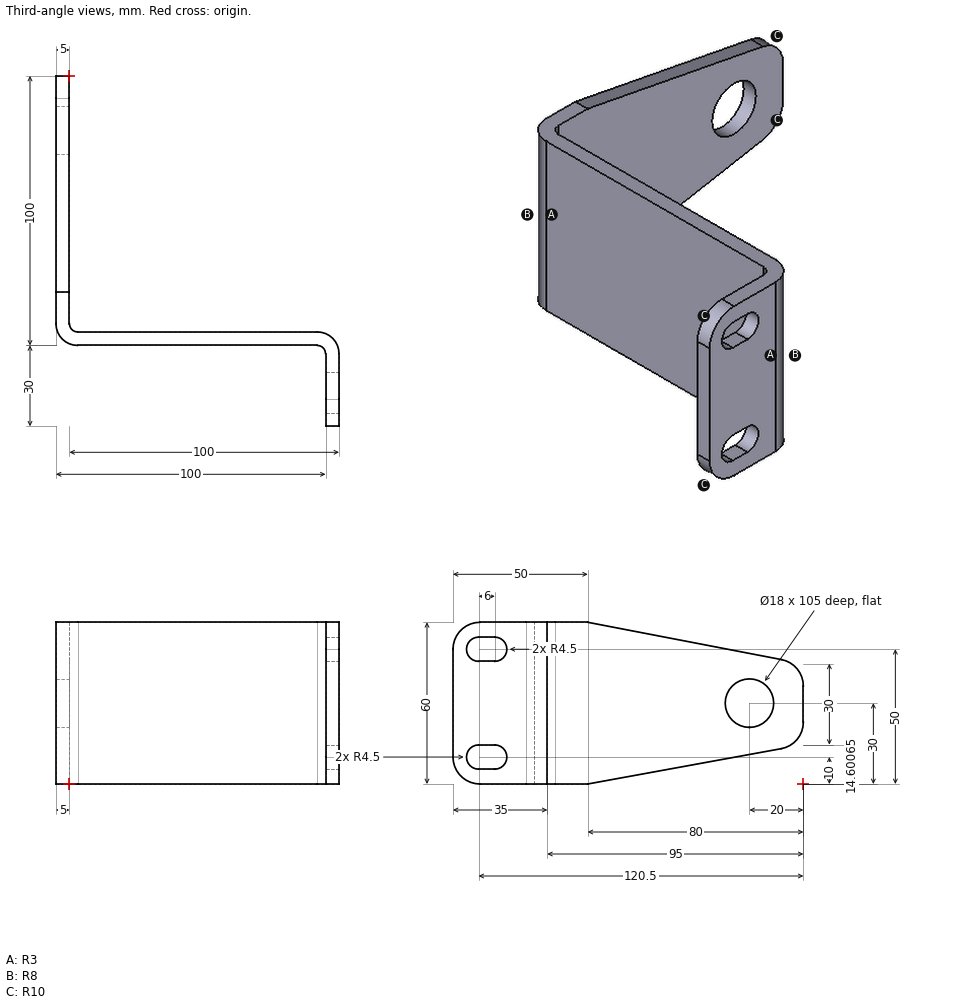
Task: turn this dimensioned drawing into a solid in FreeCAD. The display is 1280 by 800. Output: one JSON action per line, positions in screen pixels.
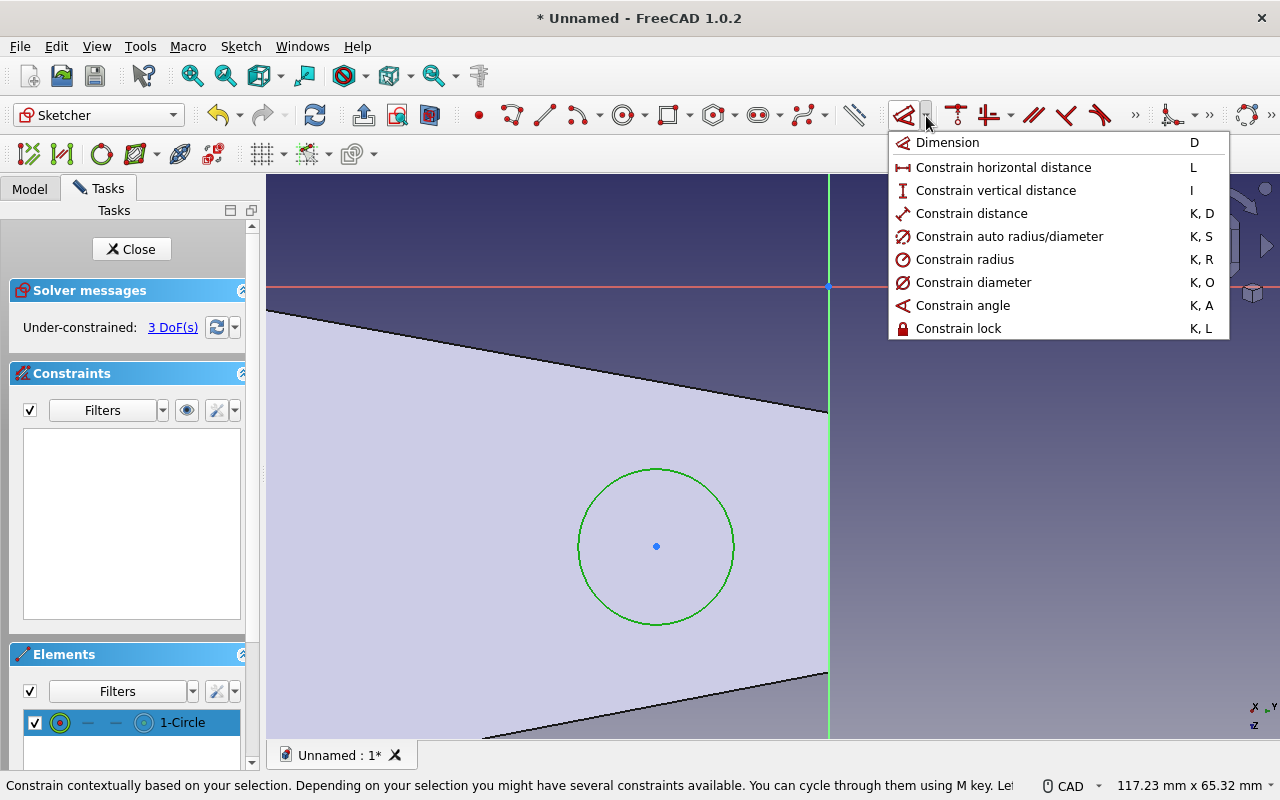
{"action": "left_click", "coordinate": [1059, 282]}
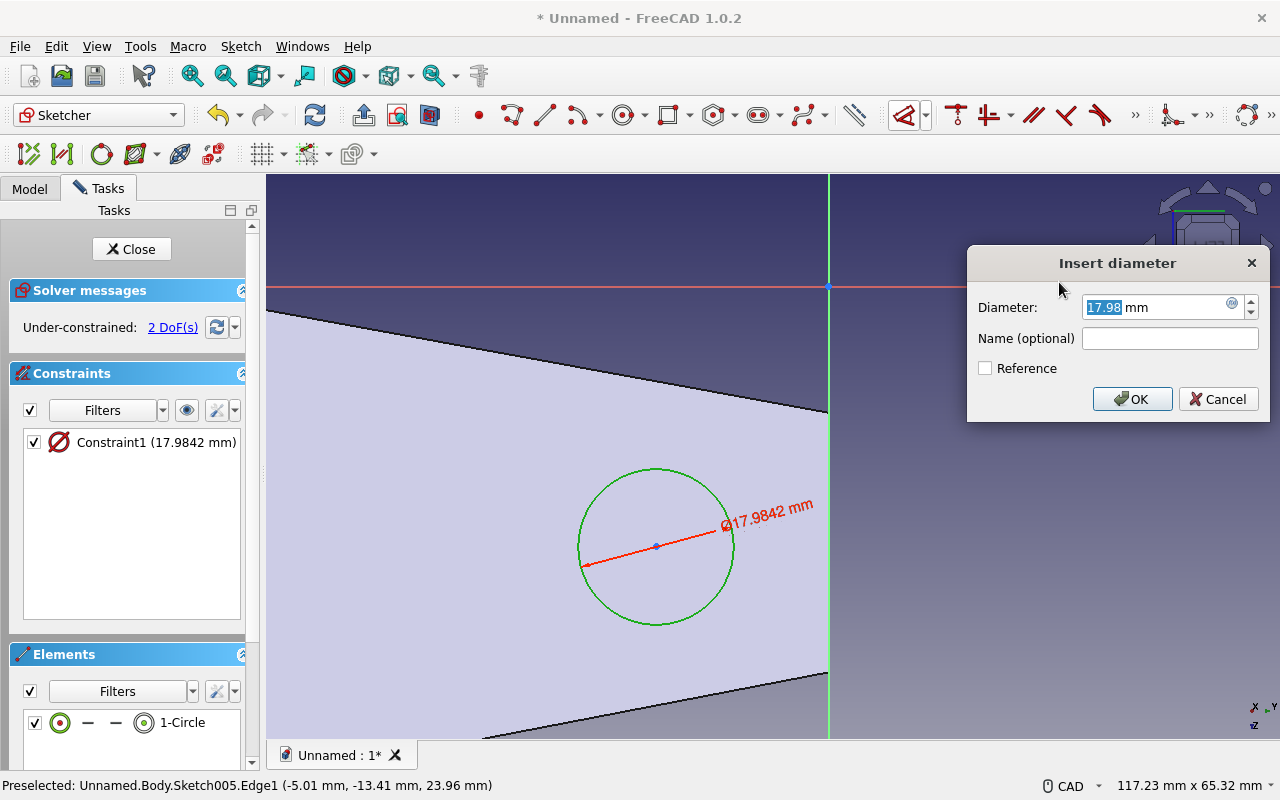
{"action": "type", "text": "18"}
{"action": "key", "text": "Return"}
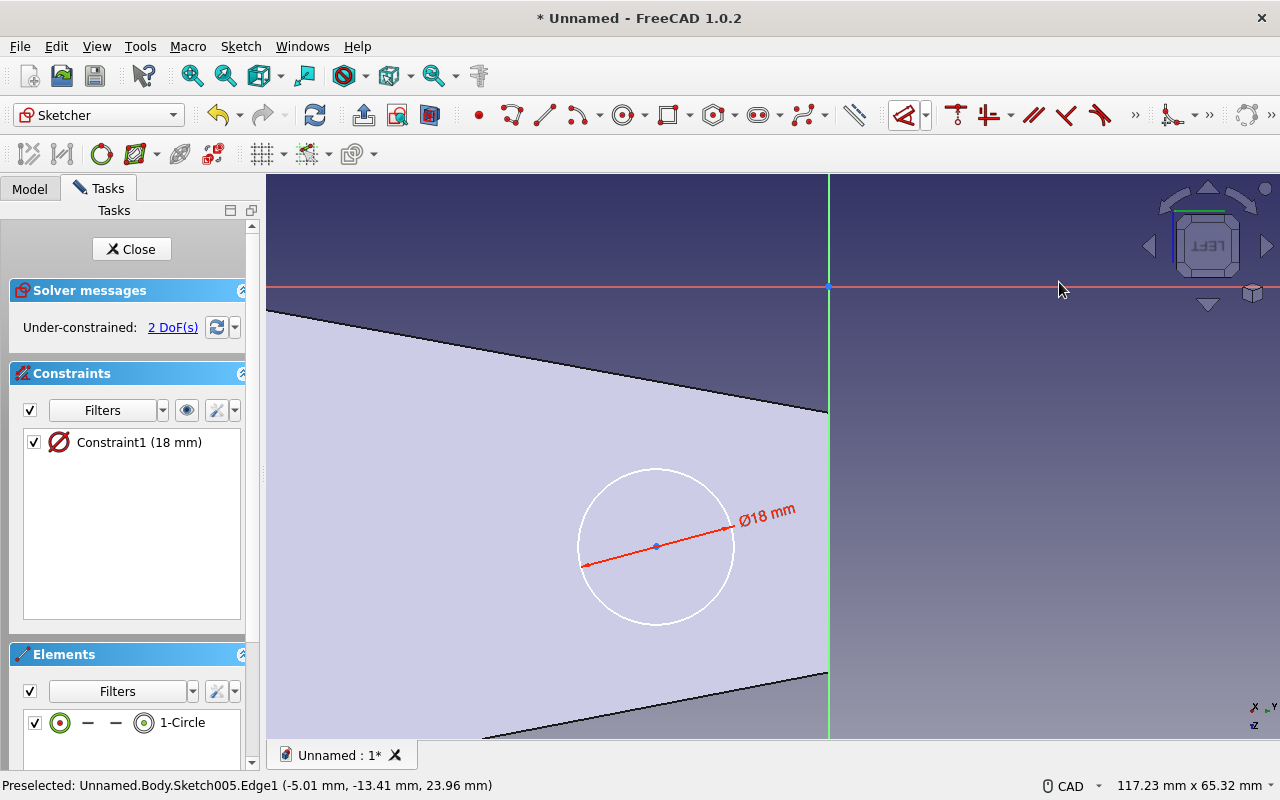
{"action": "left_click", "coordinate": [656, 547]}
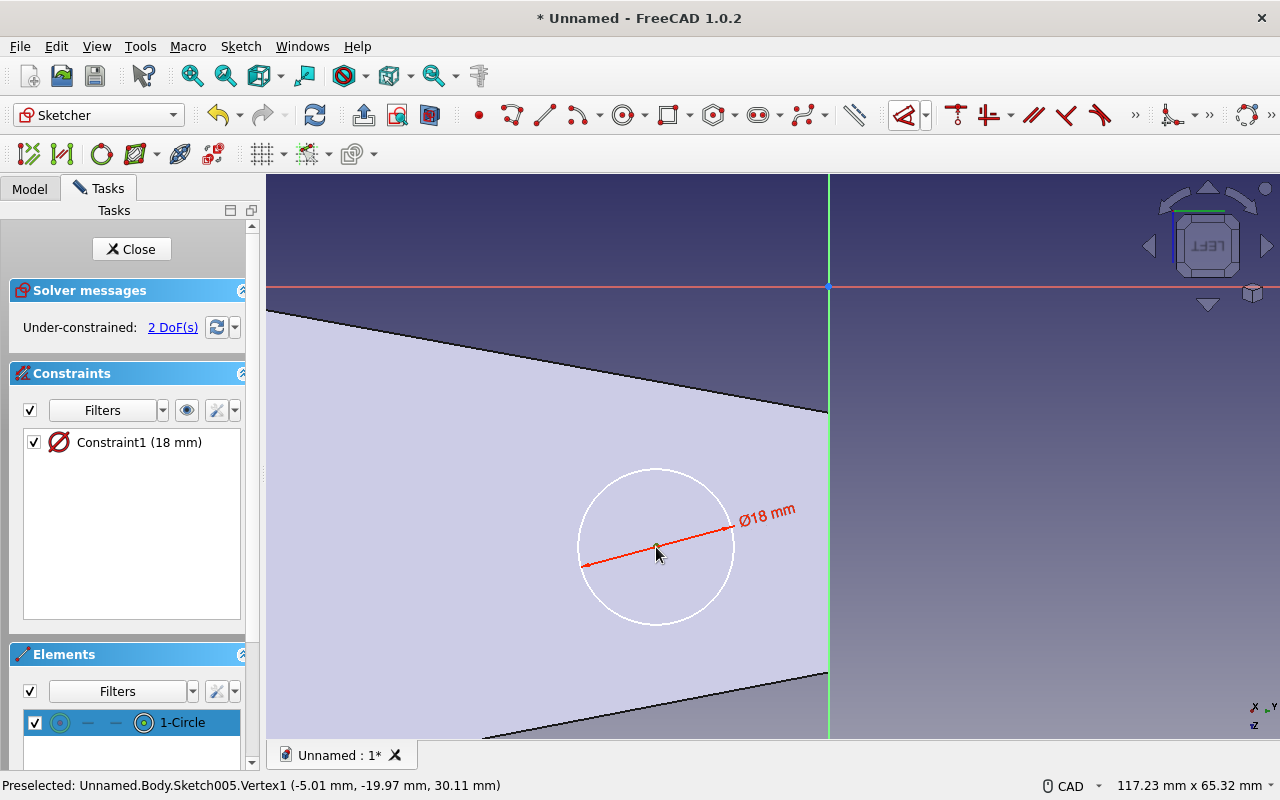
{"action": "key", "text": "l"}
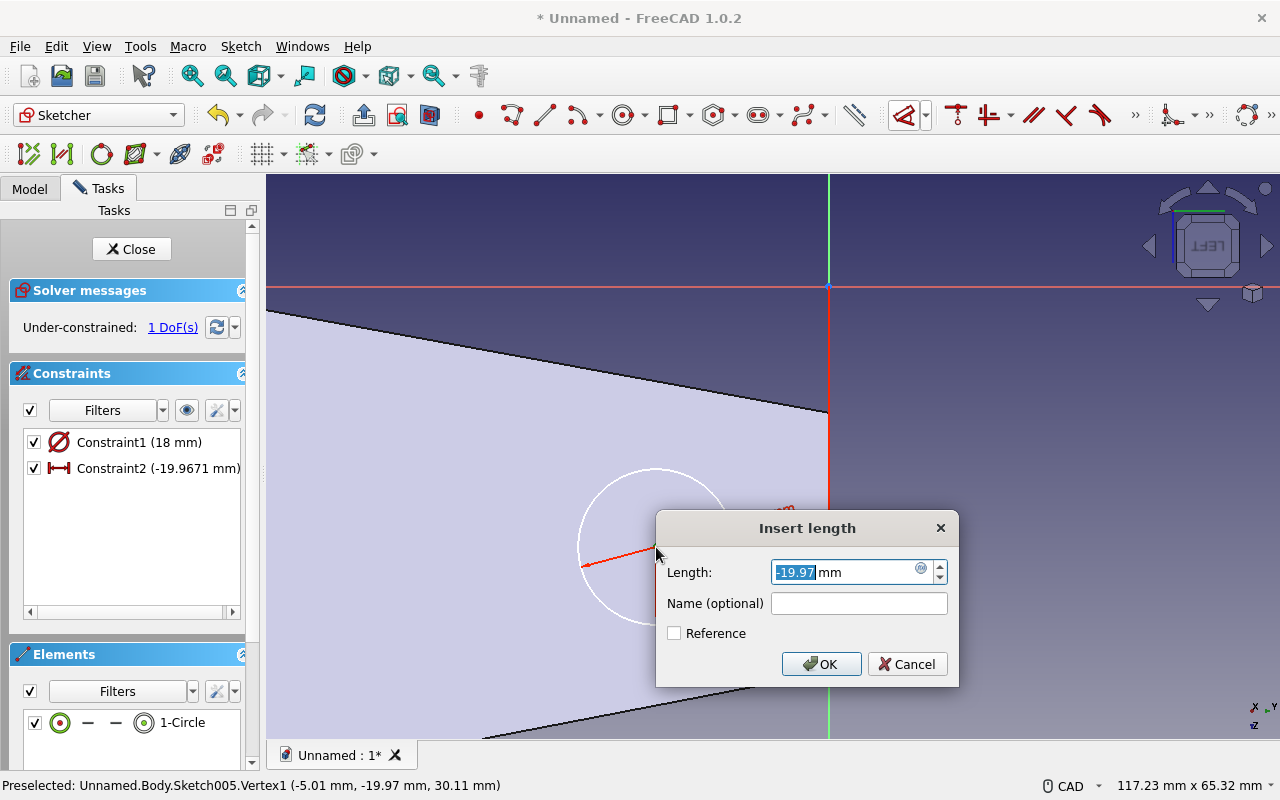
{"action": "type", "text": "-20"}
{"action": "key", "text": "Return"}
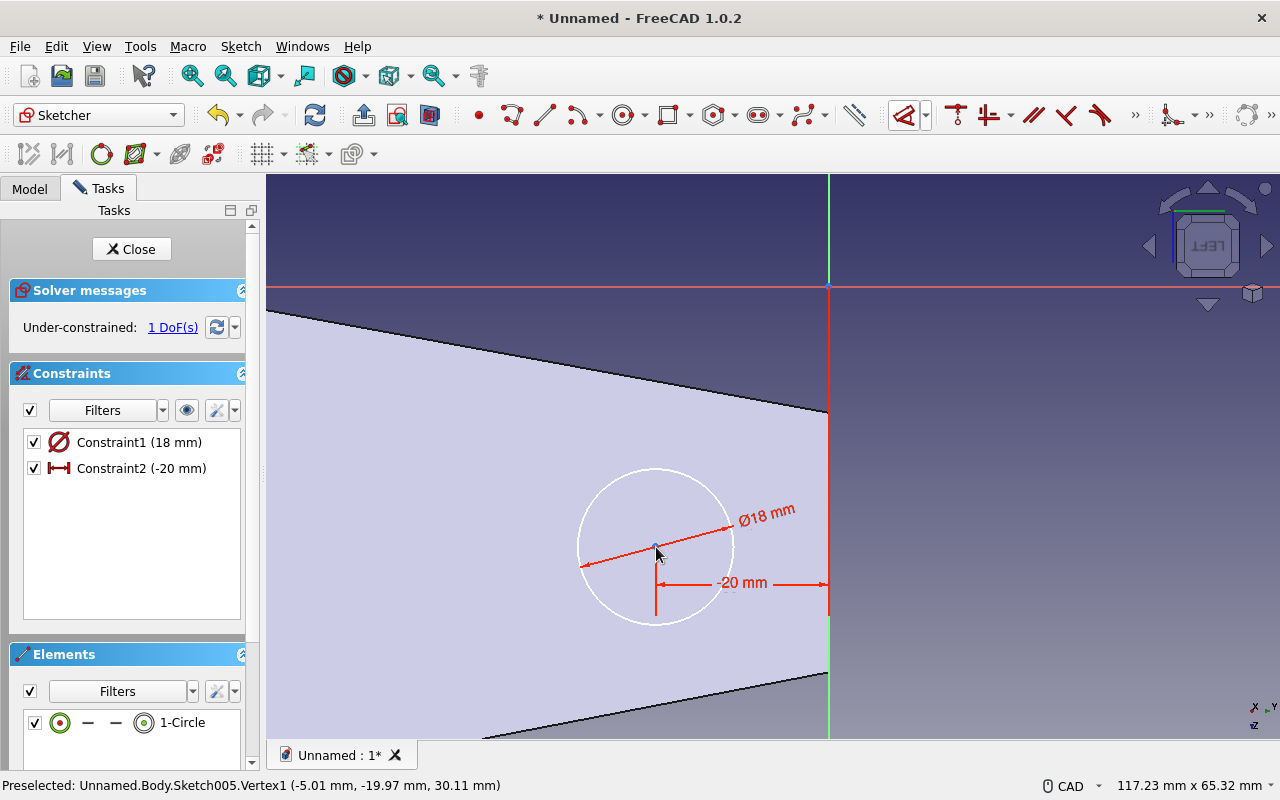
{"action": "left_click", "coordinate": [656, 547]}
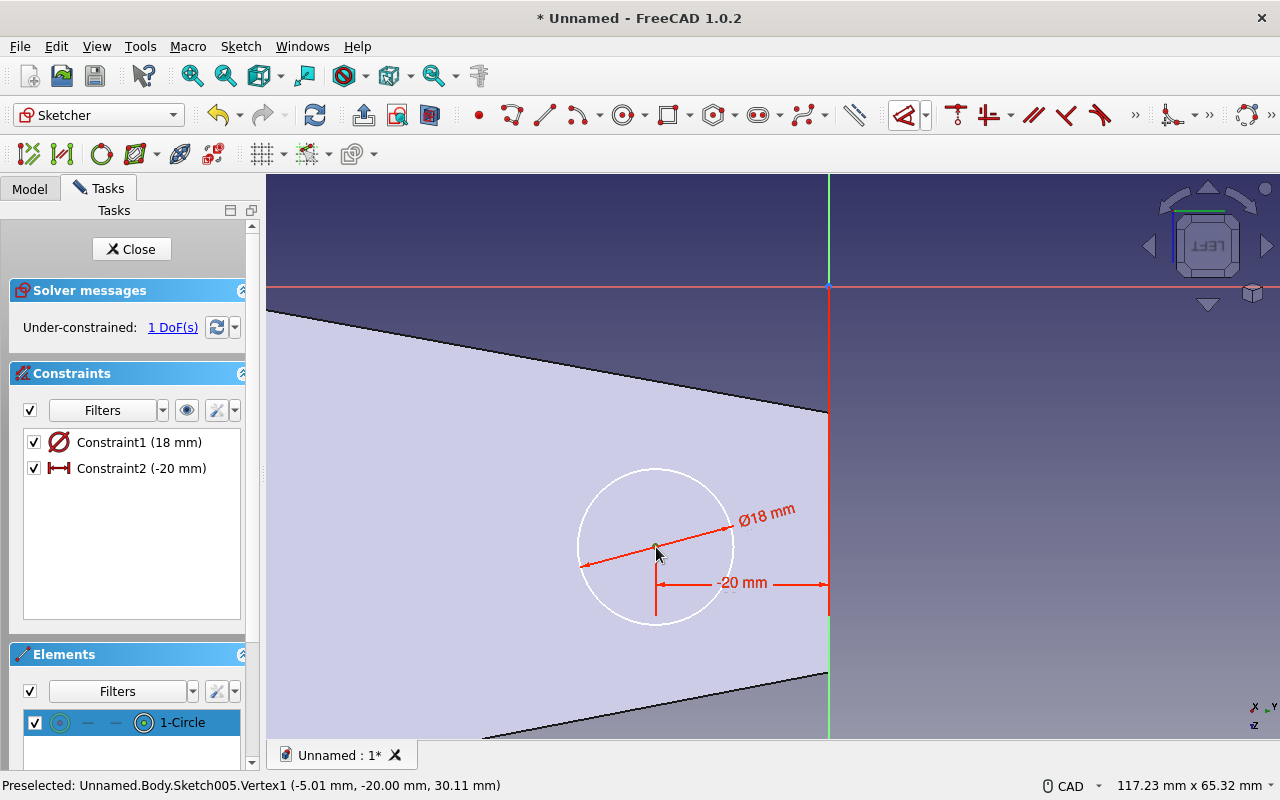
{"action": "key", "text": "i"}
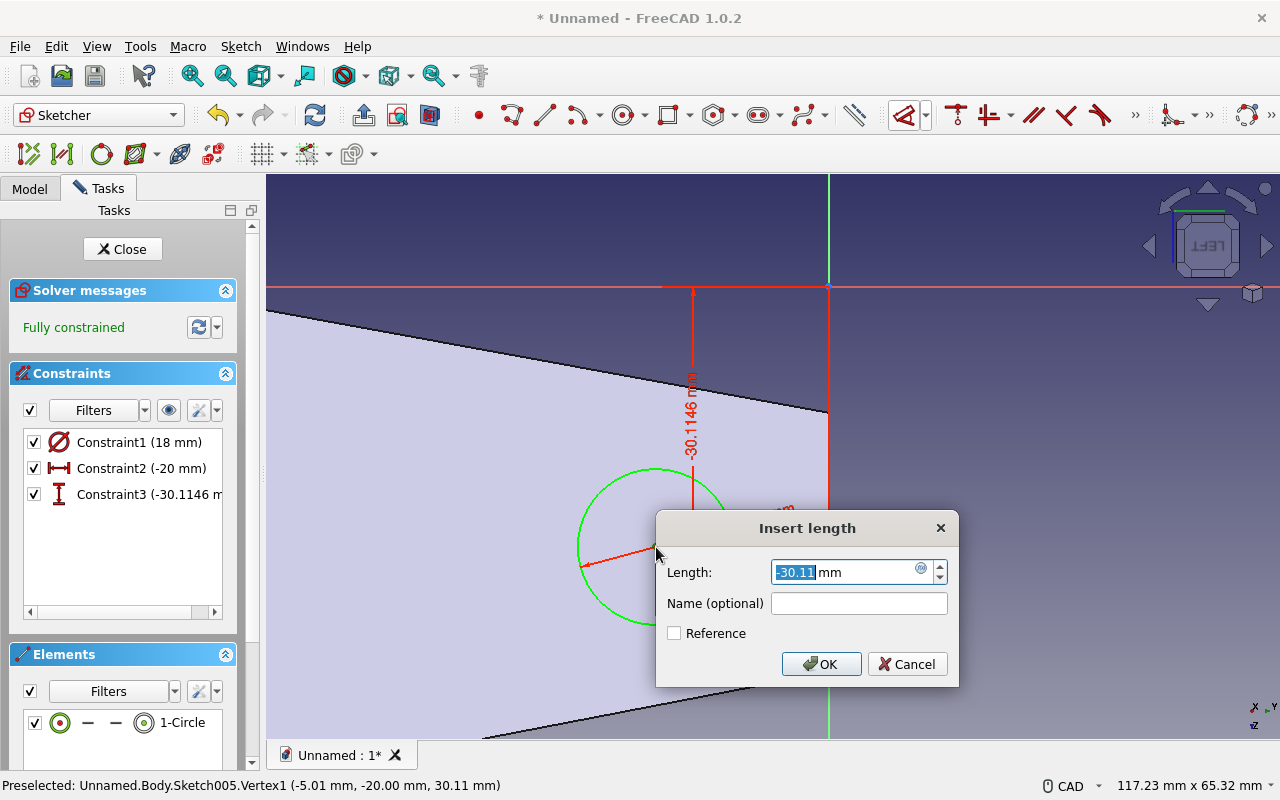
{"action": "type", "text": "-30"}
{"action": "key", "text": "Return"}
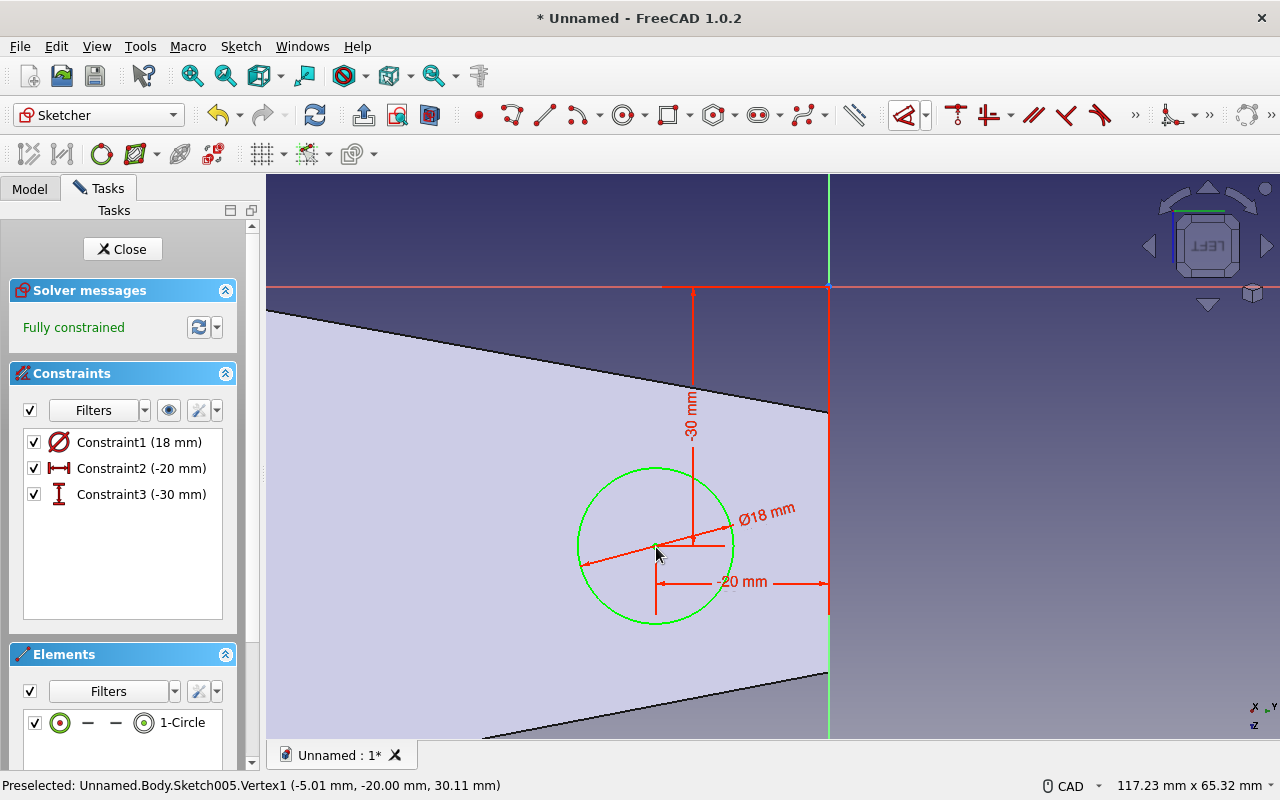
{"action": "left_click", "coordinate": [123, 249]}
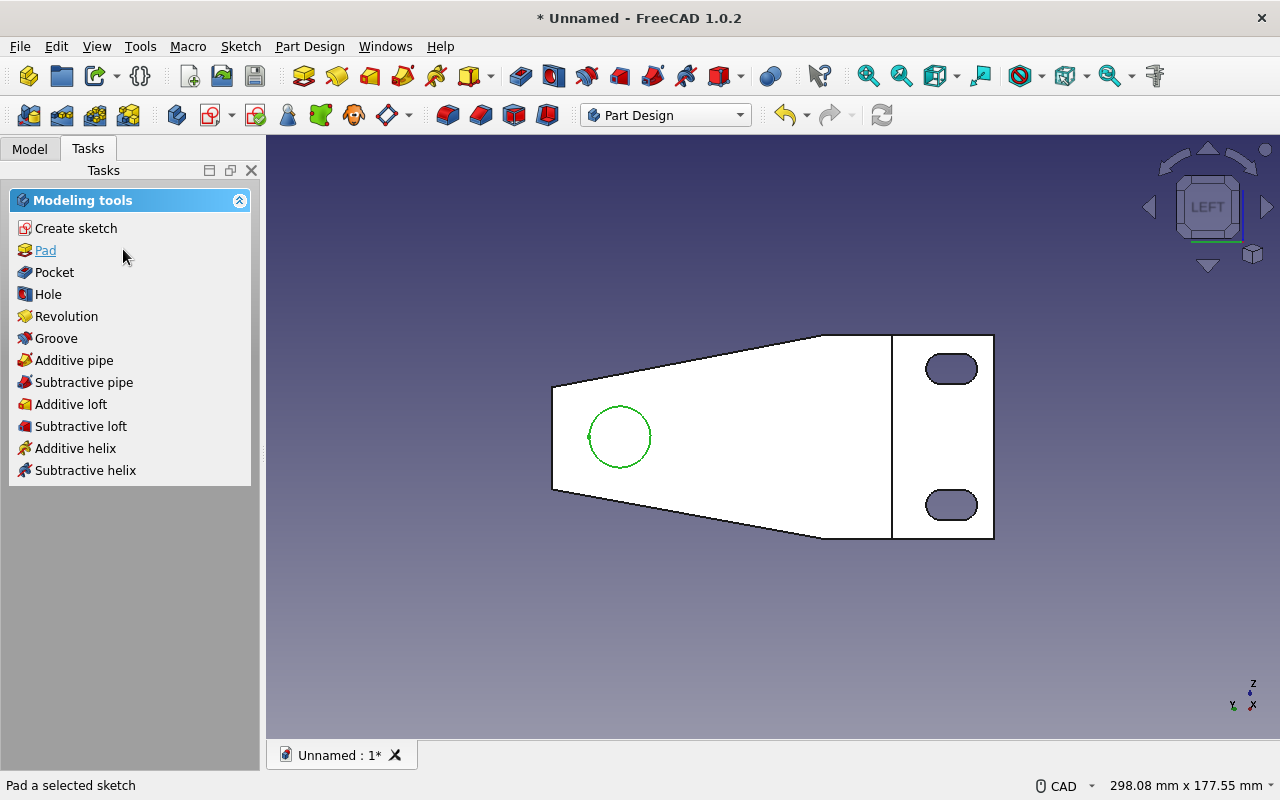
{"action": "left_click", "coordinate": [554, 76]}